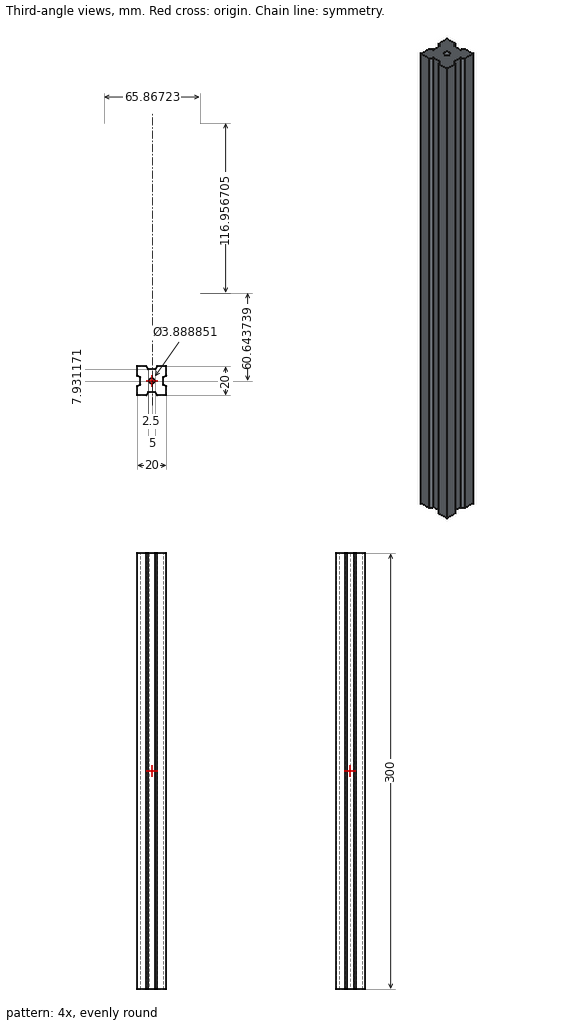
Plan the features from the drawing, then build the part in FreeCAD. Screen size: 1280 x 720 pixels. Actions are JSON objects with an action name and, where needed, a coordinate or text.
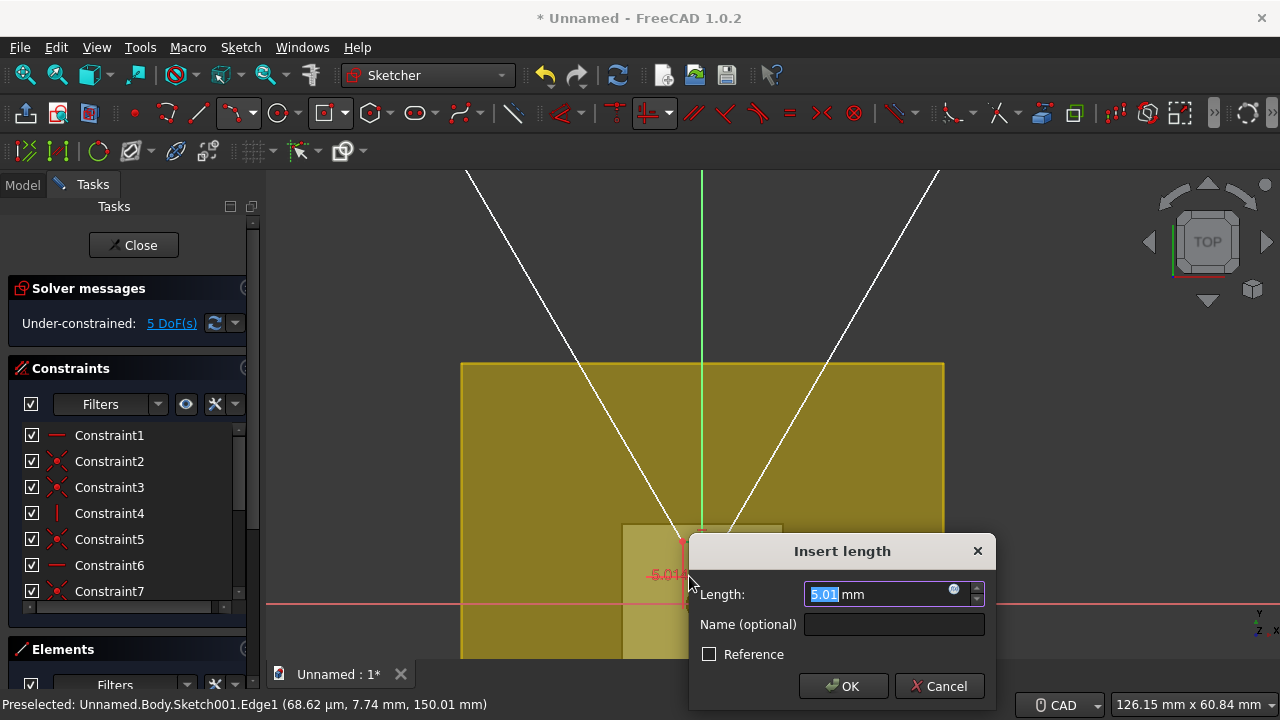
{"action": "type", "text": "5"}
{"action": "key", "text": "Return"}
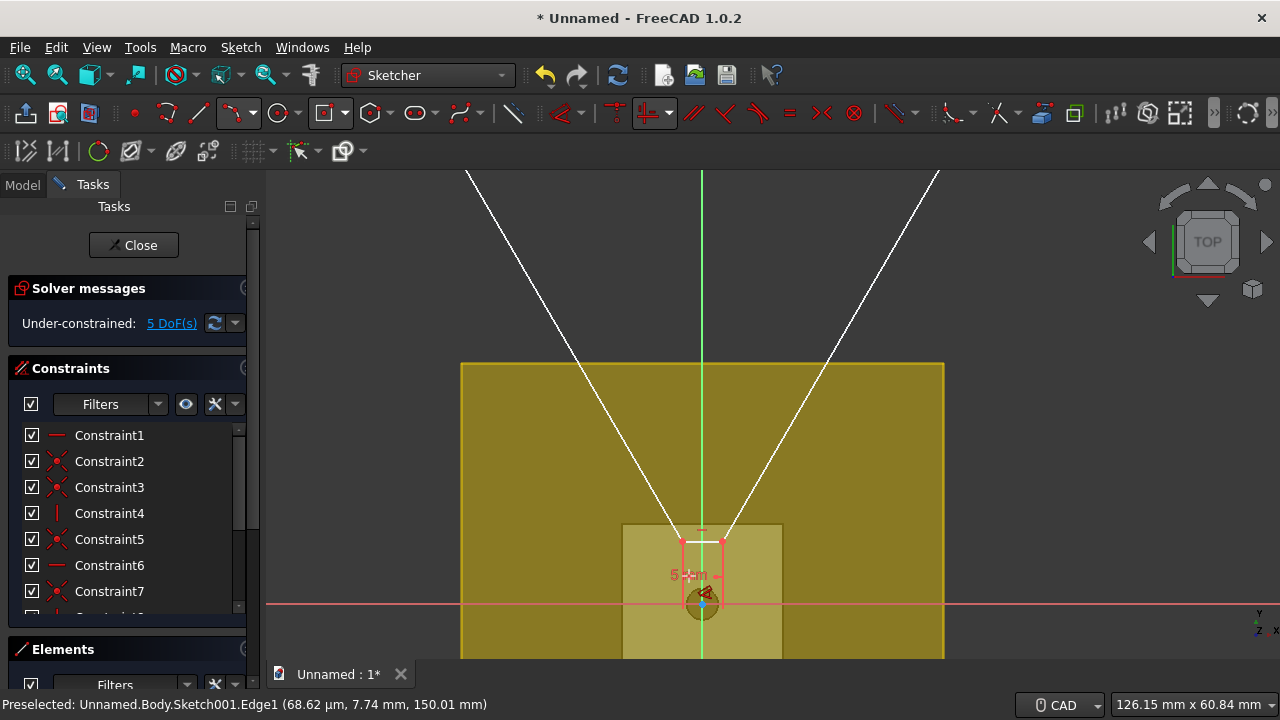
{"action": "scroll", "coordinate": [683, 542], "scroll_direction": "up", "scroll_amount": 4}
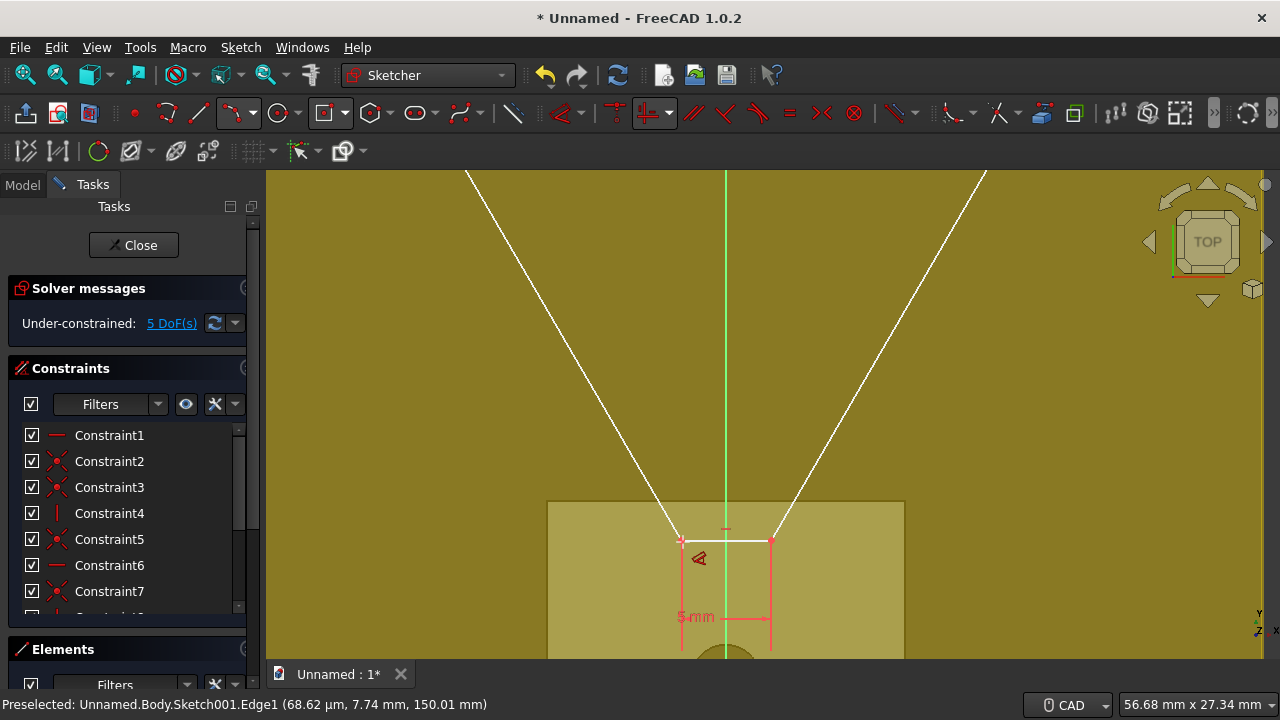
{"action": "left_click", "coordinate": [682, 541]}
{"action": "left_click", "coordinate": [704, 507]}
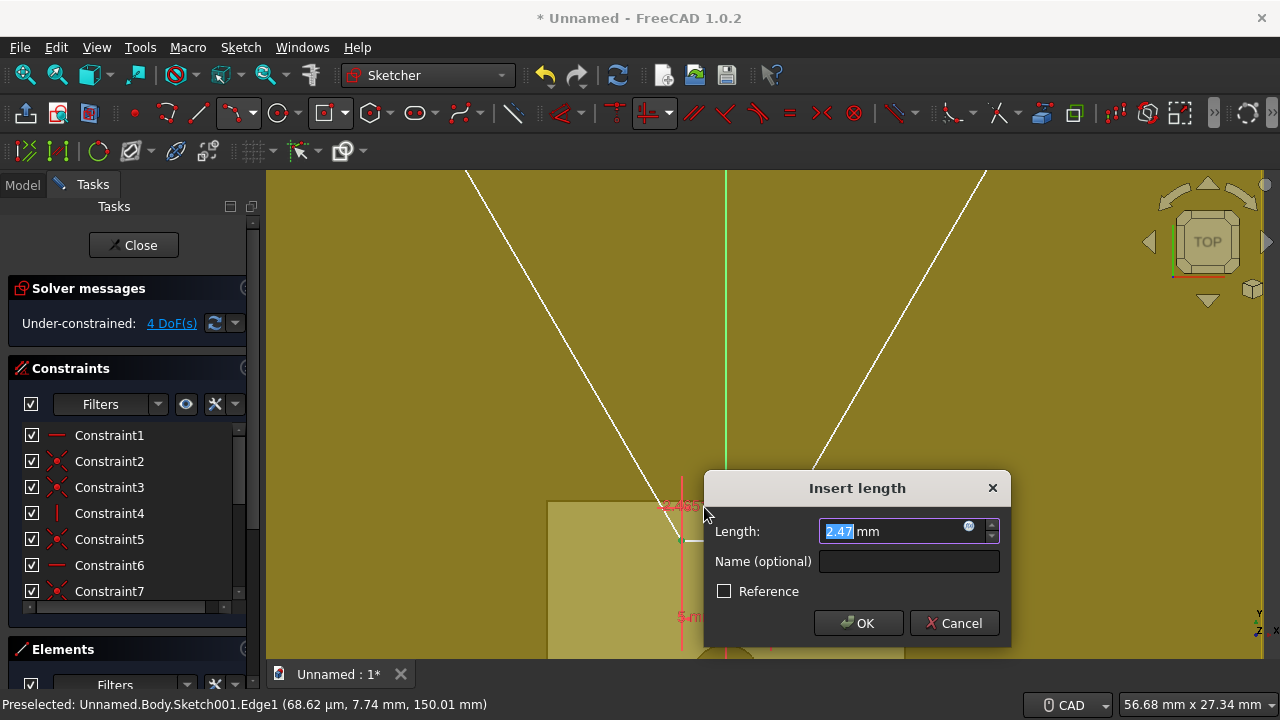
{"action": "type", "text": "2.5"}
{"action": "key", "text": "Return"}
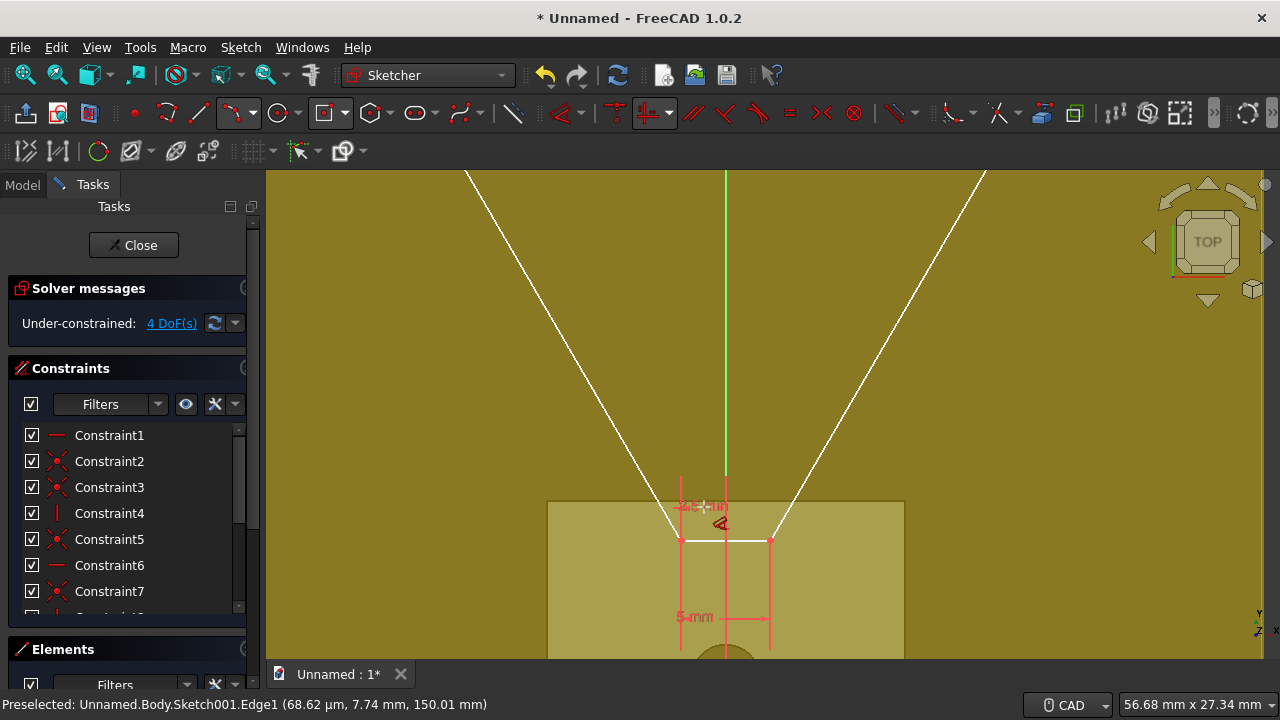
{"action": "scroll", "coordinate": [702, 547], "scroll_direction": "down", "scroll_amount": 12}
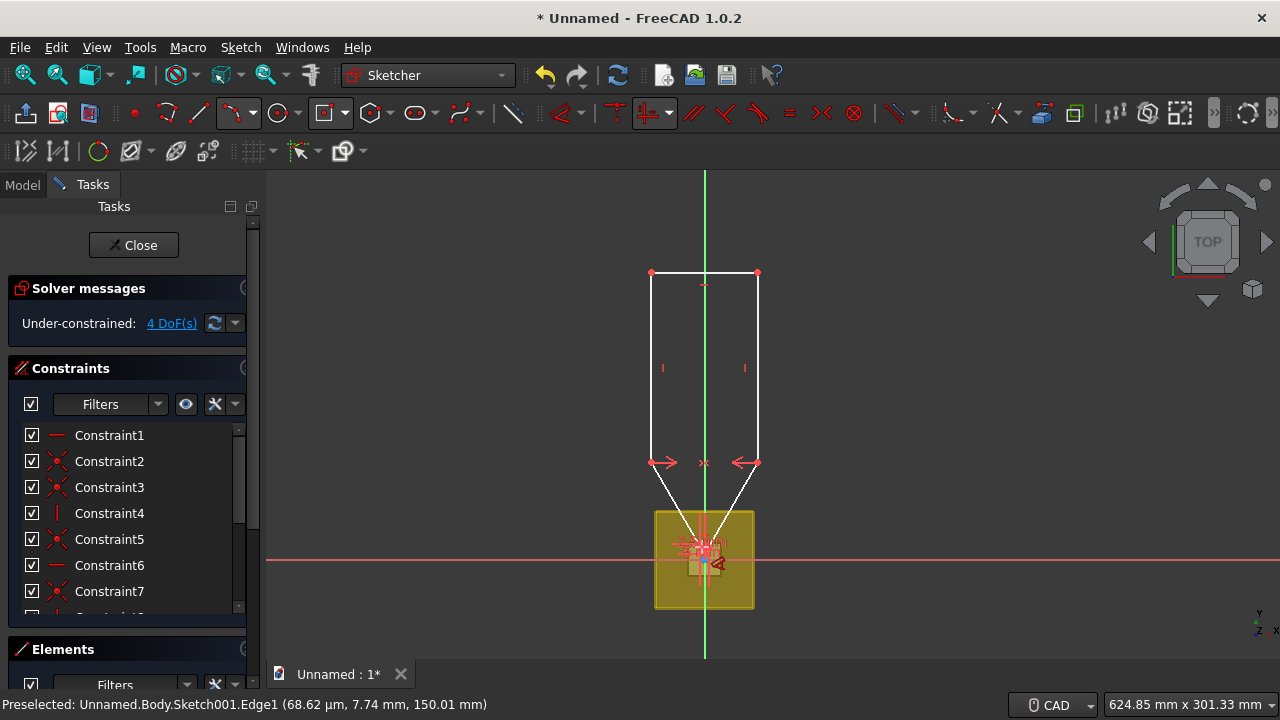
{"action": "left_click", "coordinate": [726, 273]}
{"action": "left_click", "coordinate": [680, 239]}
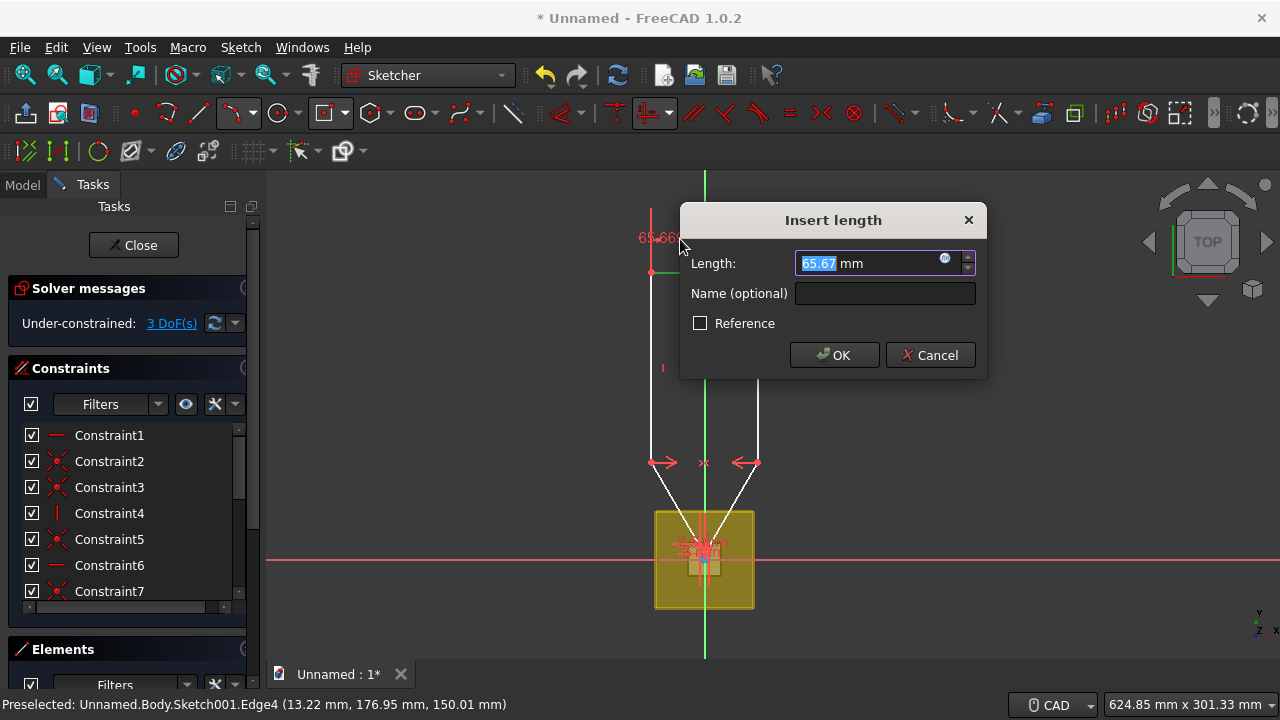
{"action": "type", "text": "65.86723"}
{"action": "key", "text": "Return"}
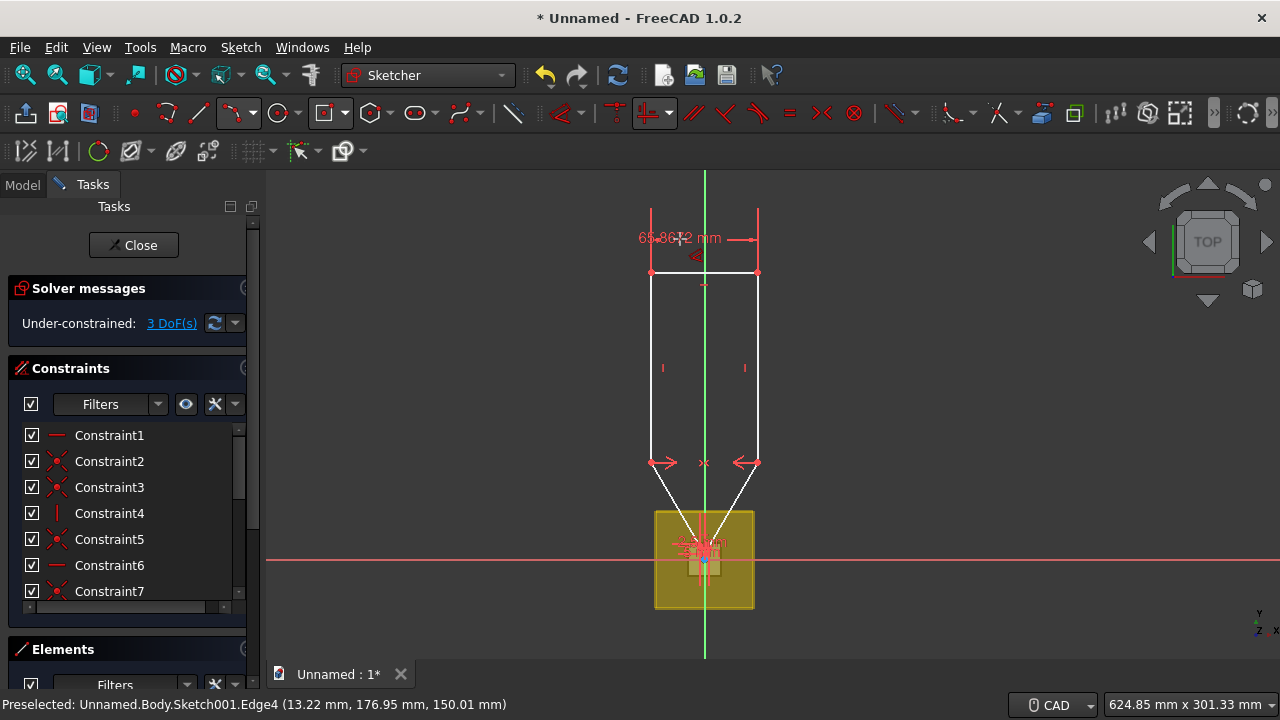
{"action": "scroll", "coordinate": [700, 547], "scroll_direction": "up", "scroll_amount": 6}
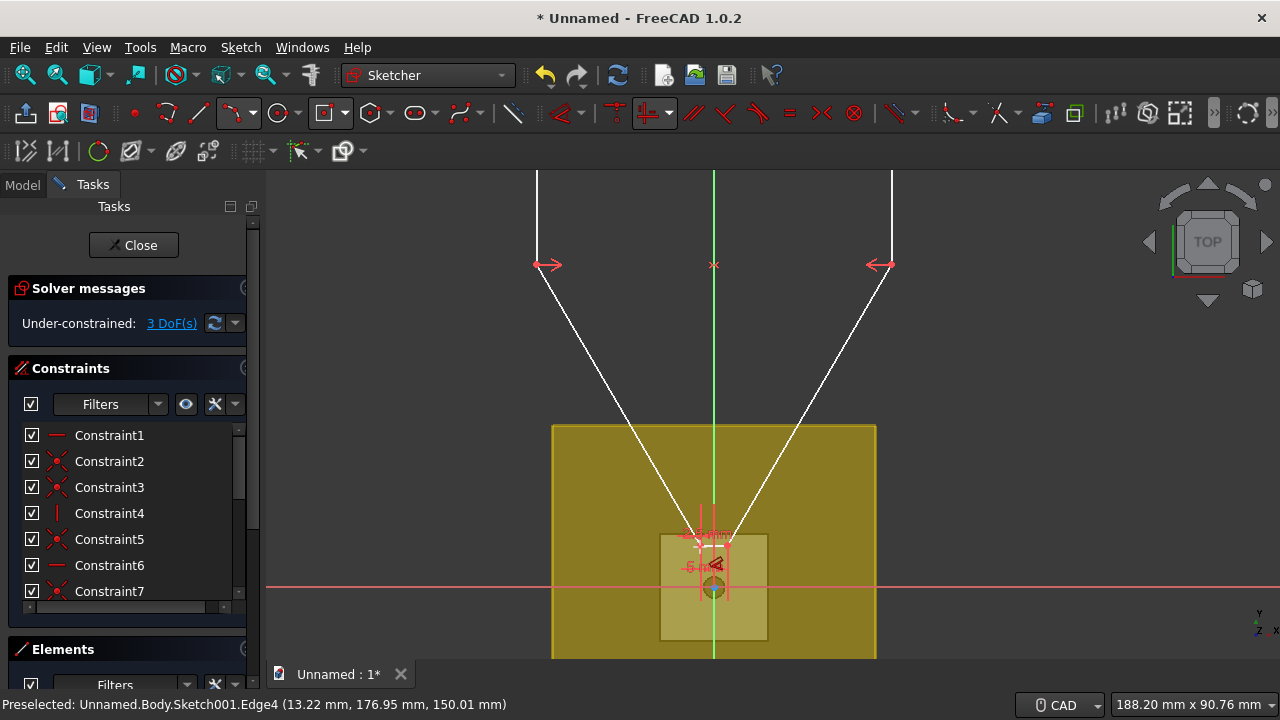
{"action": "left_click", "coordinate": [701, 546]}
{"action": "left_click", "coordinate": [619, 567]}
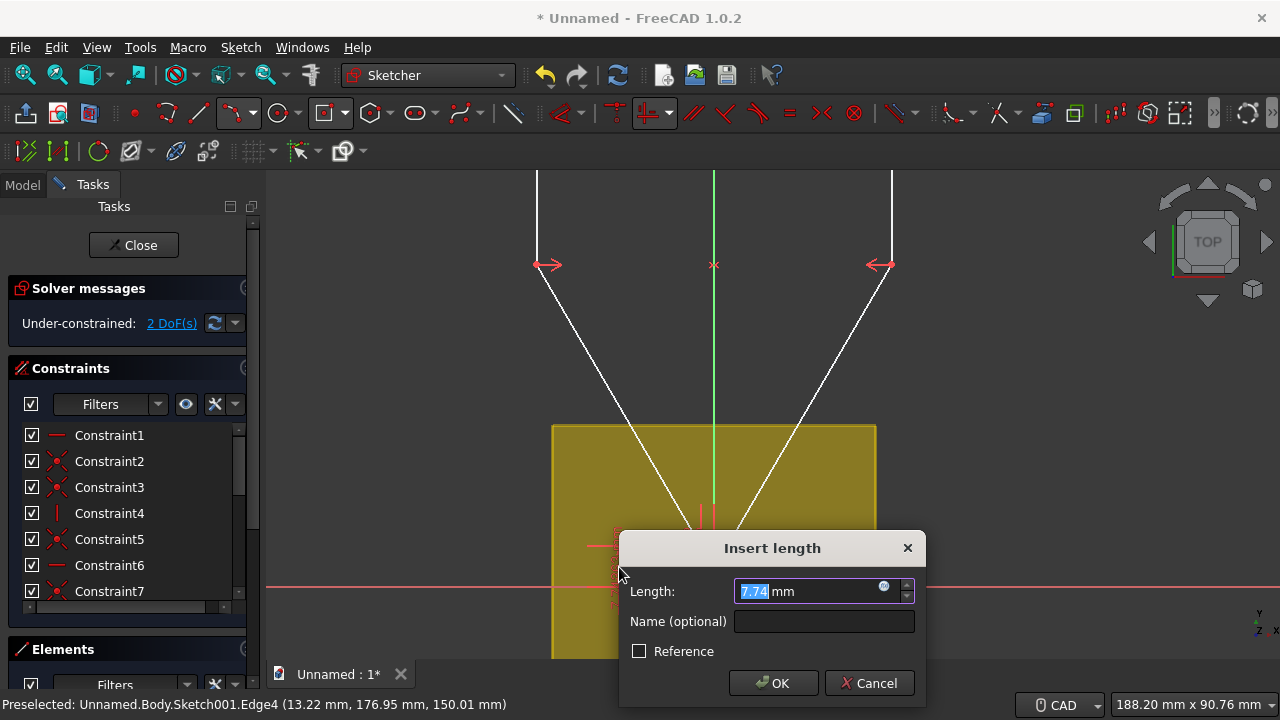
{"action": "type", "text": "7.931171"}
{"action": "key", "text": "Return"}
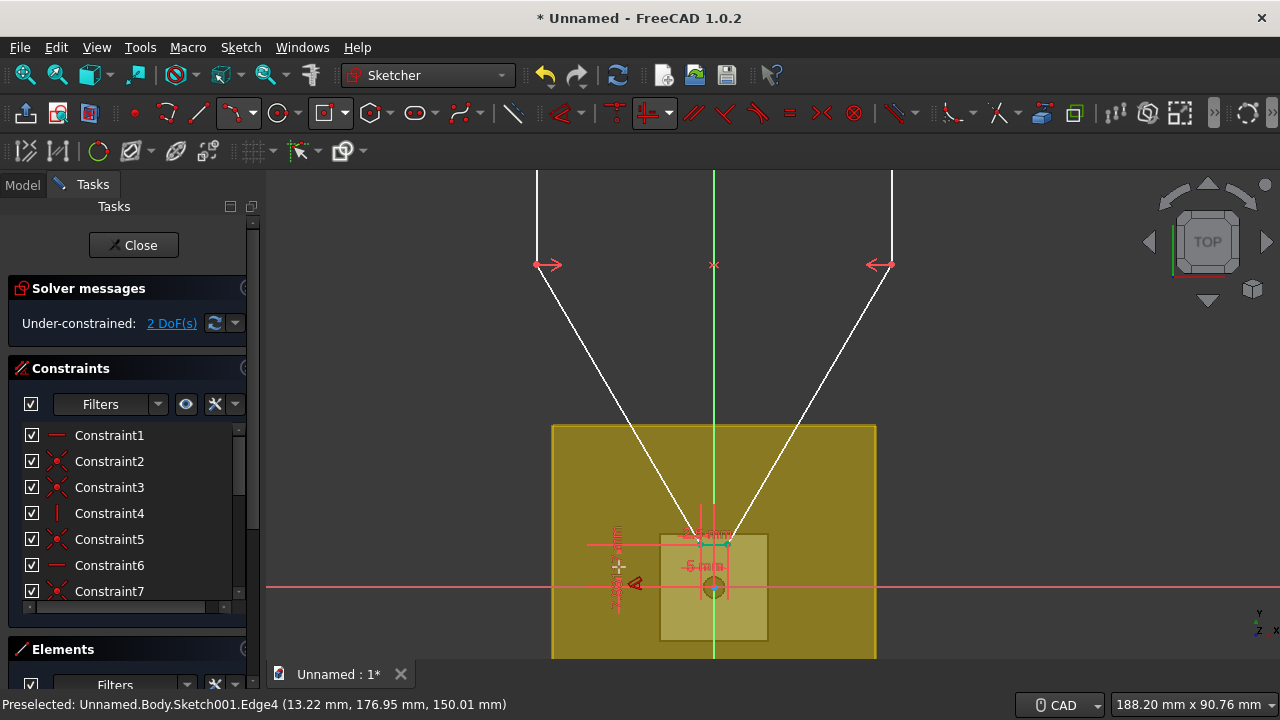
{"action": "scroll", "coordinate": [700, 546], "scroll_direction": "down", "scroll_amount": 6}